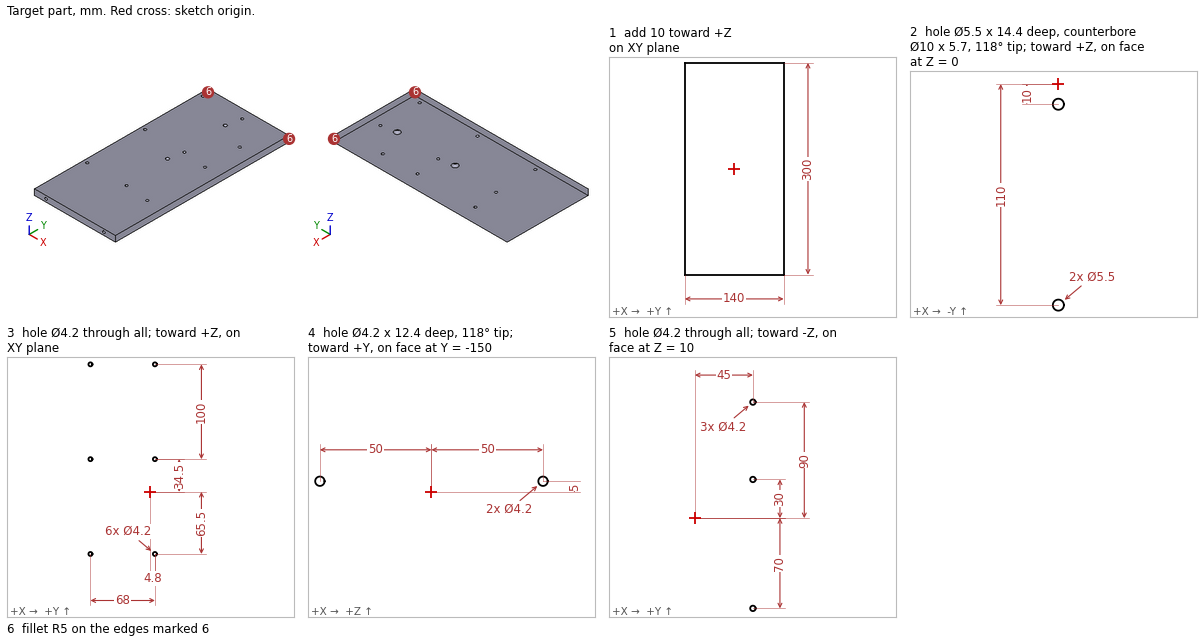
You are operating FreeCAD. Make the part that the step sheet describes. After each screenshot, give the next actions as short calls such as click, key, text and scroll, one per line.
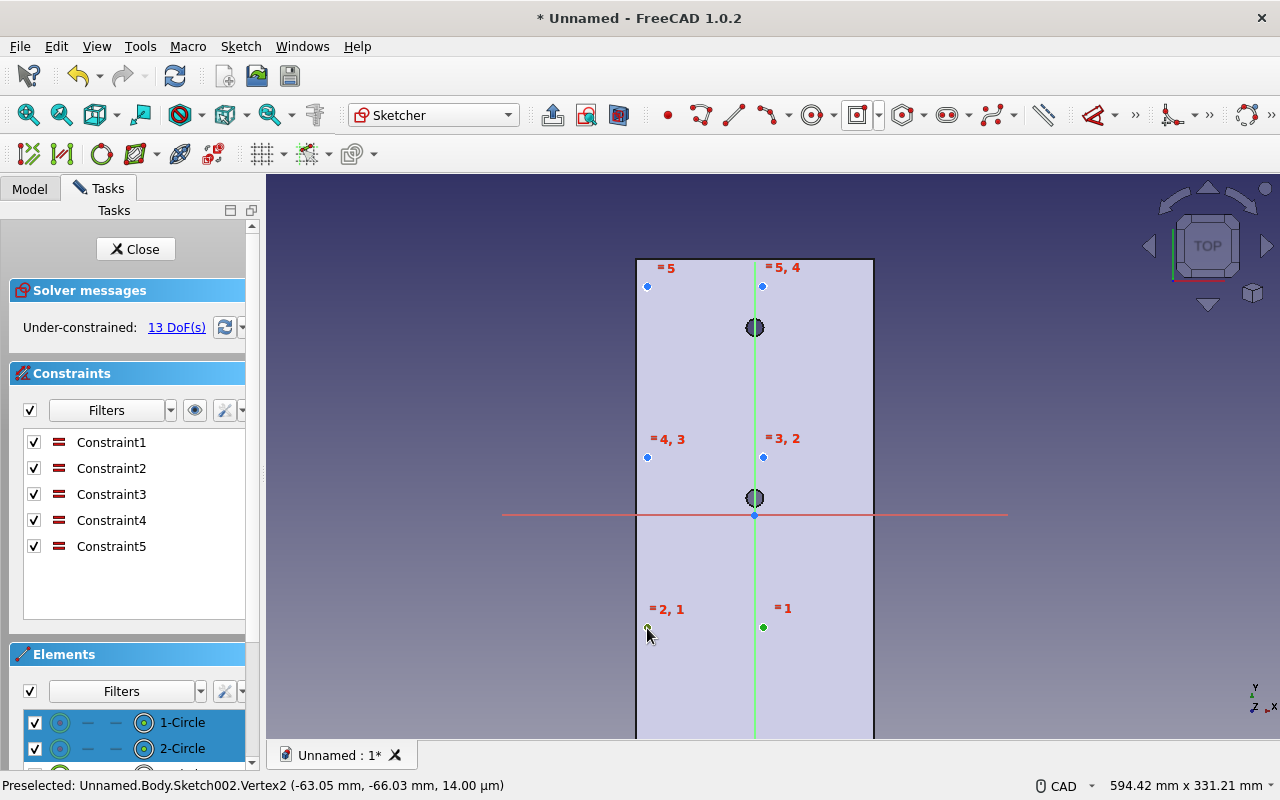
key(h)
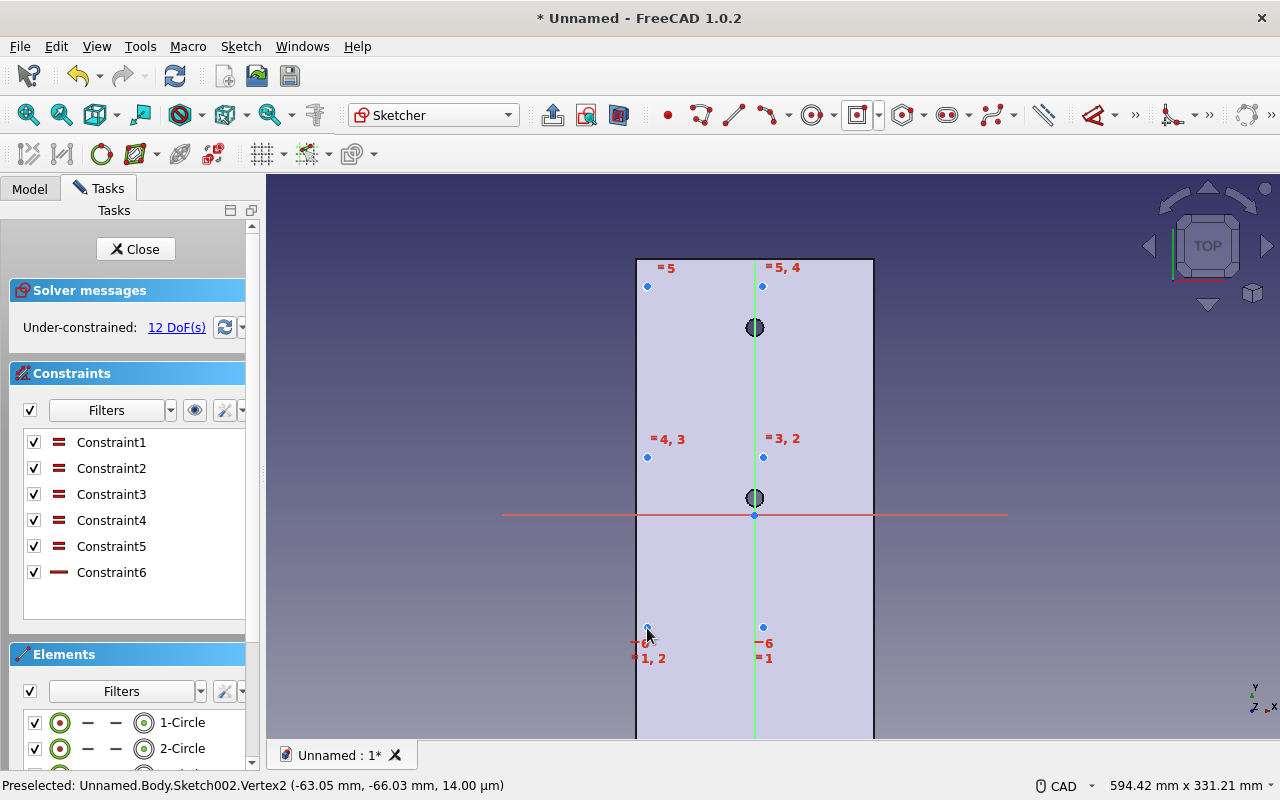
click(763, 627)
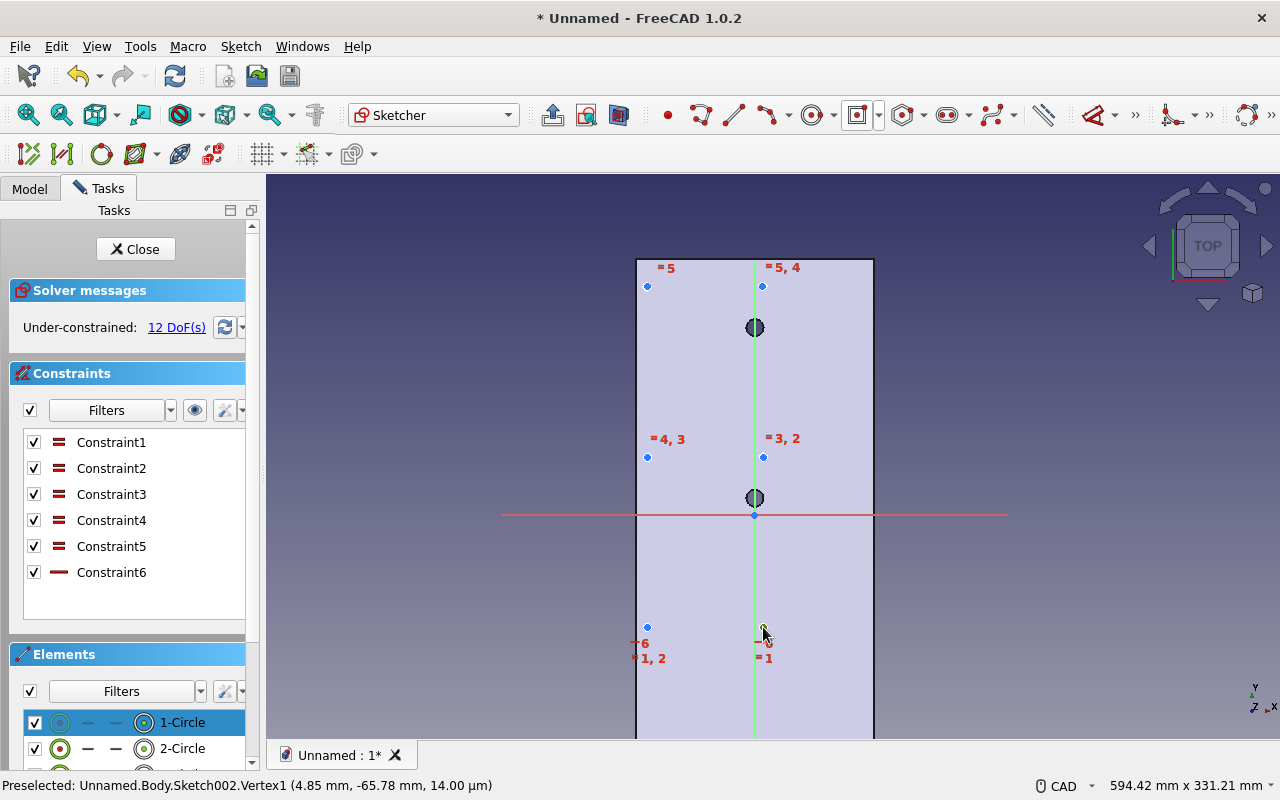
click(763, 457)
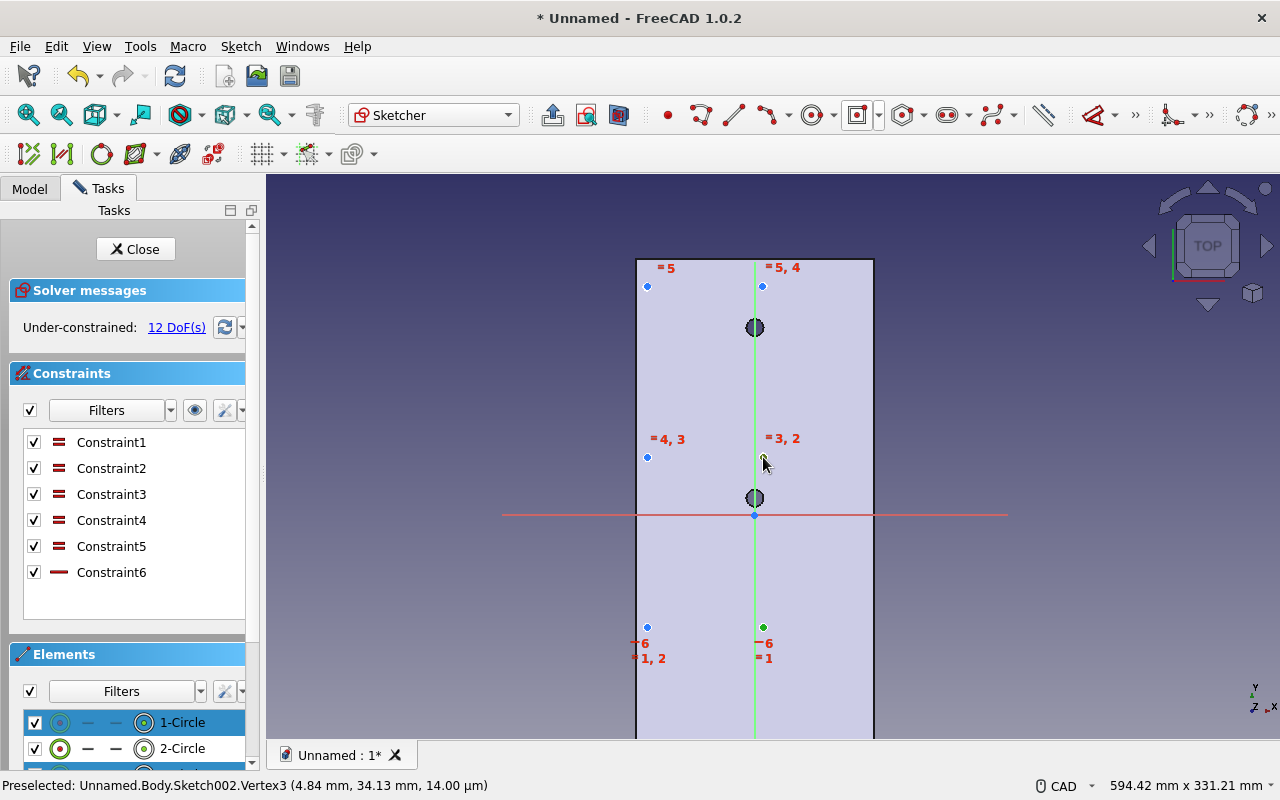
key(v)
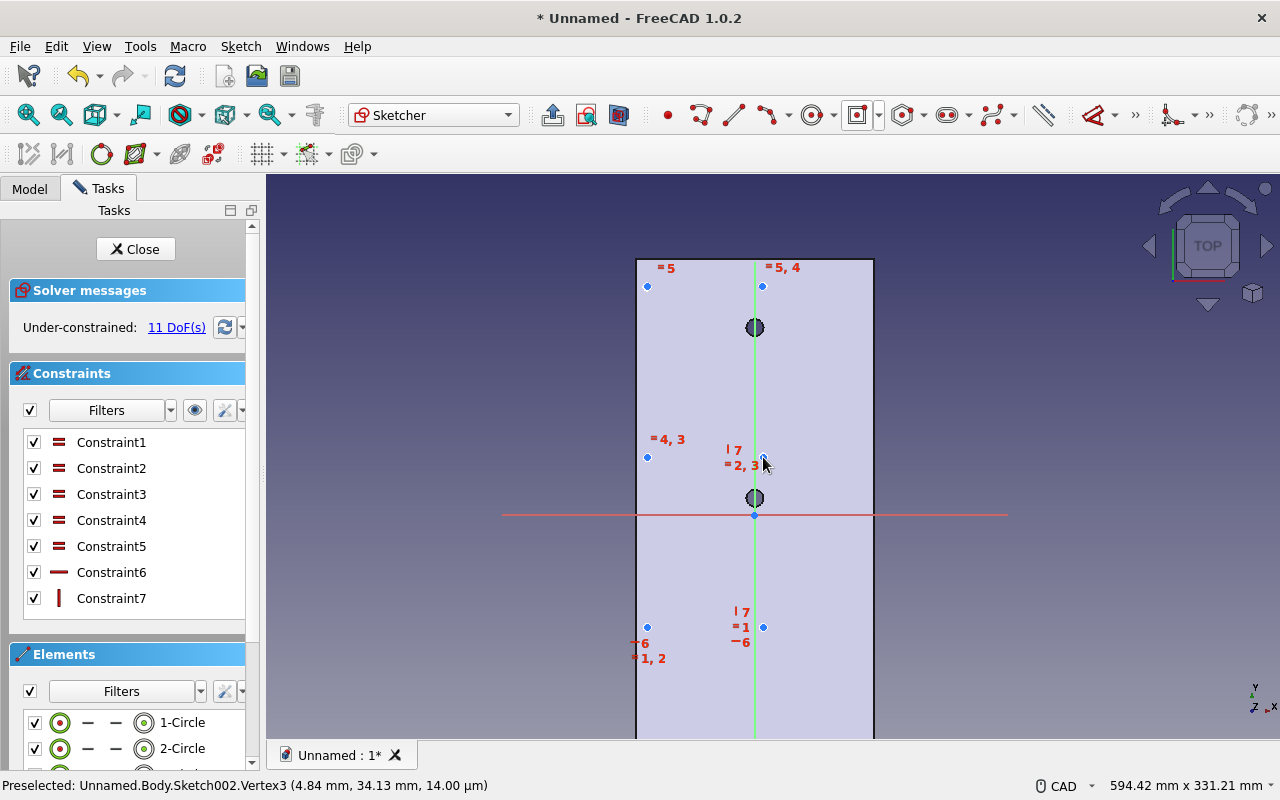
click(647, 627)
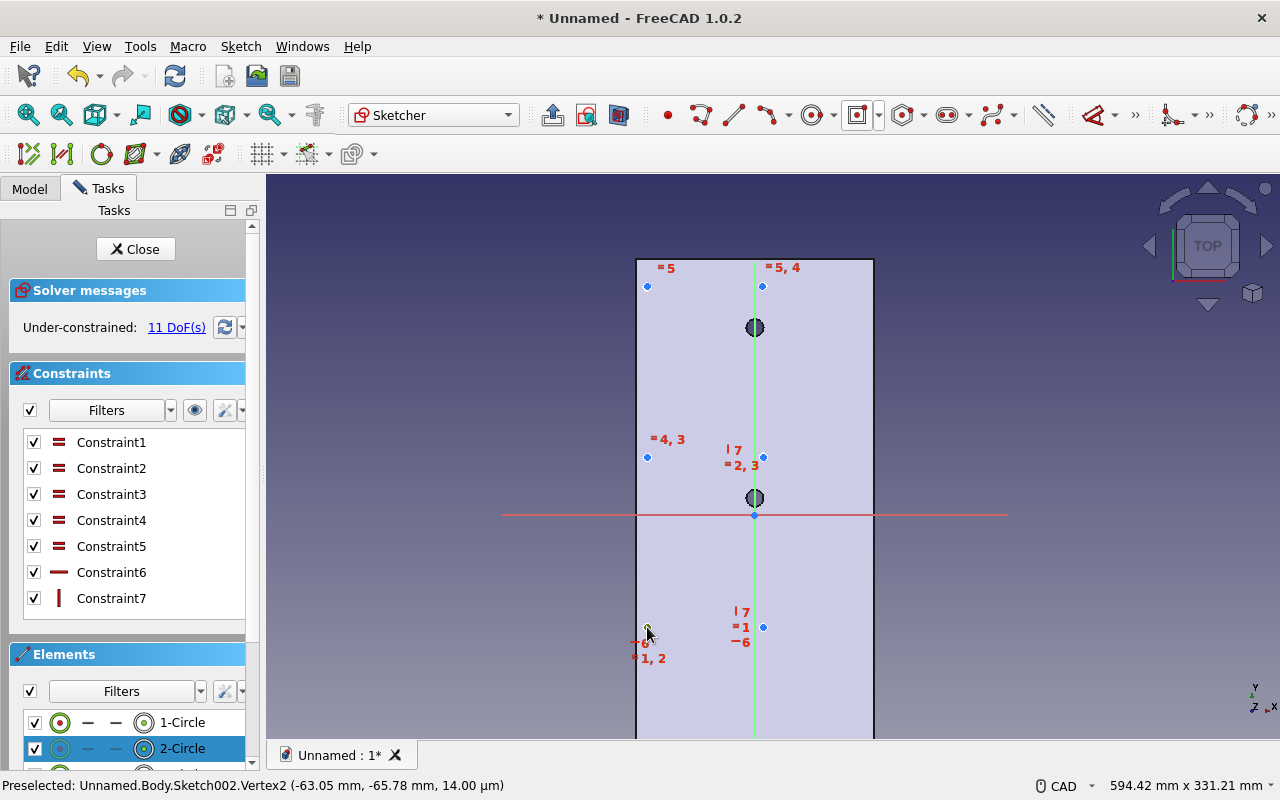
click(648, 458)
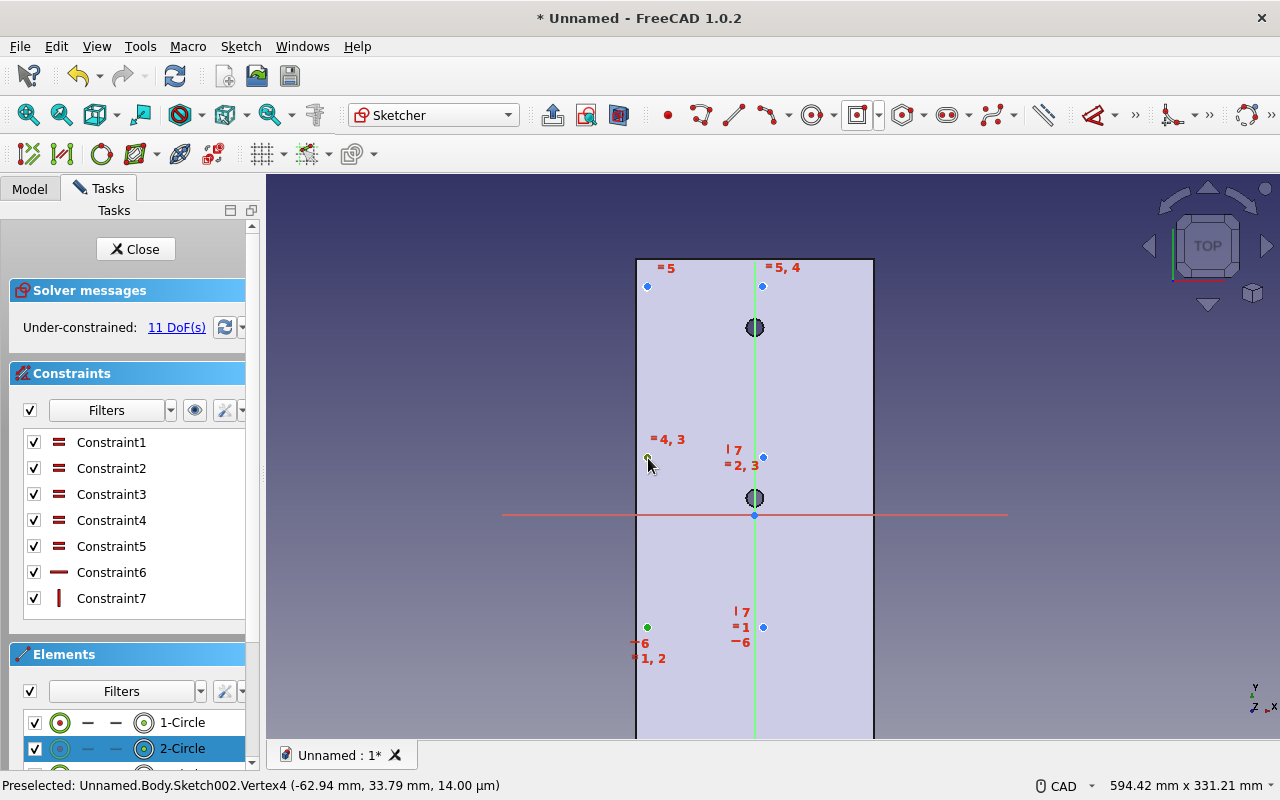
key(v)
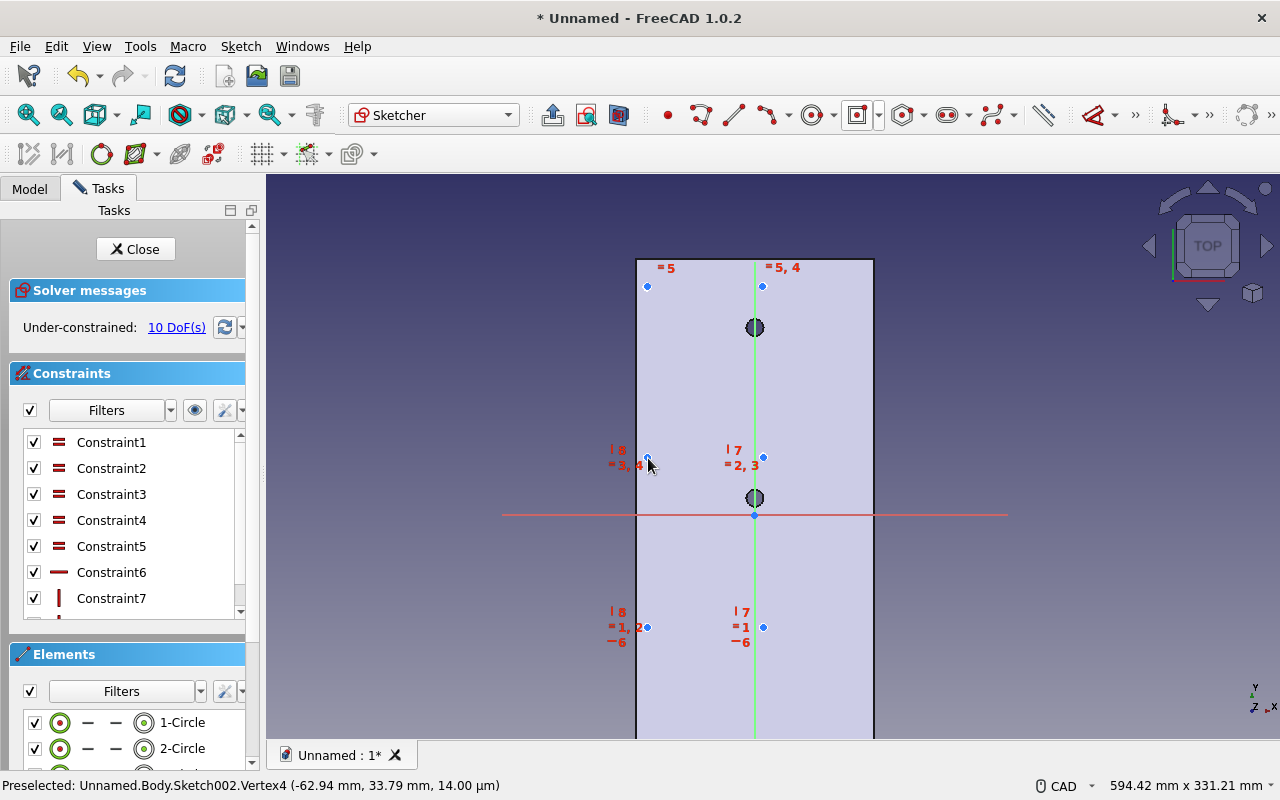
click(763, 457)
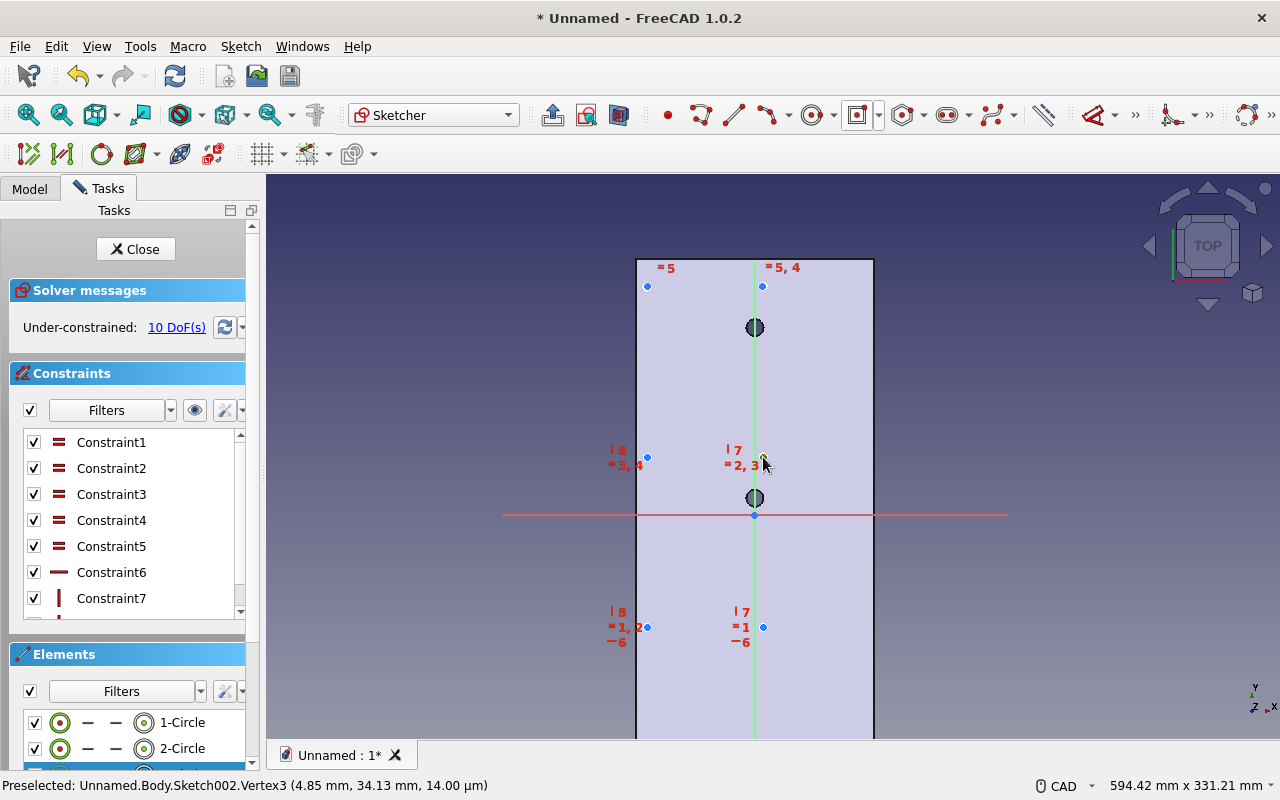
click(647, 458)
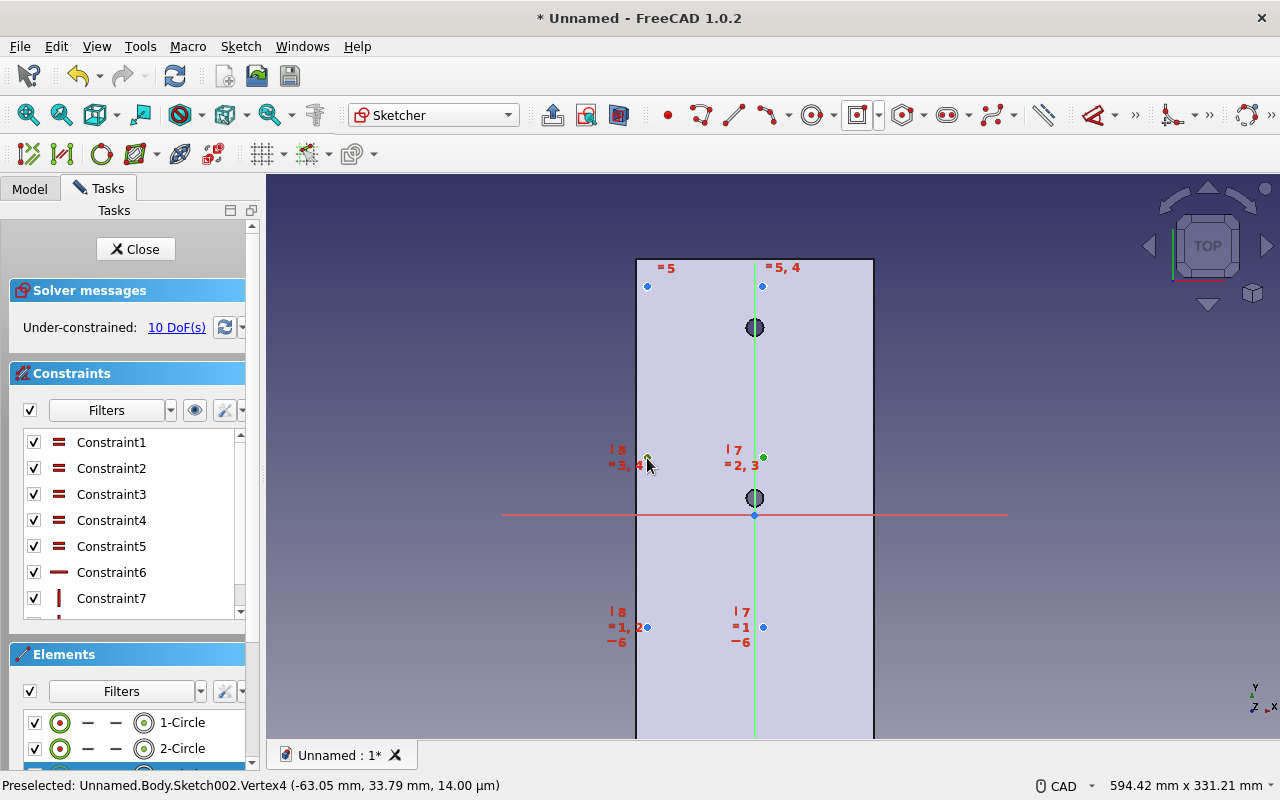
key(h)